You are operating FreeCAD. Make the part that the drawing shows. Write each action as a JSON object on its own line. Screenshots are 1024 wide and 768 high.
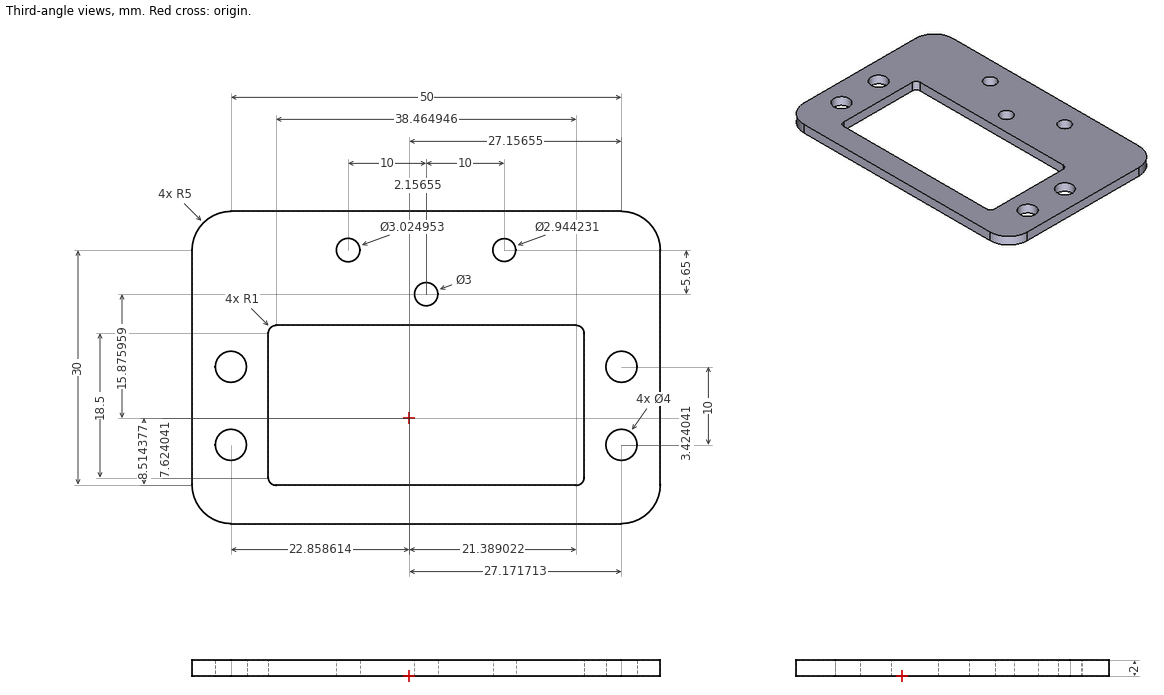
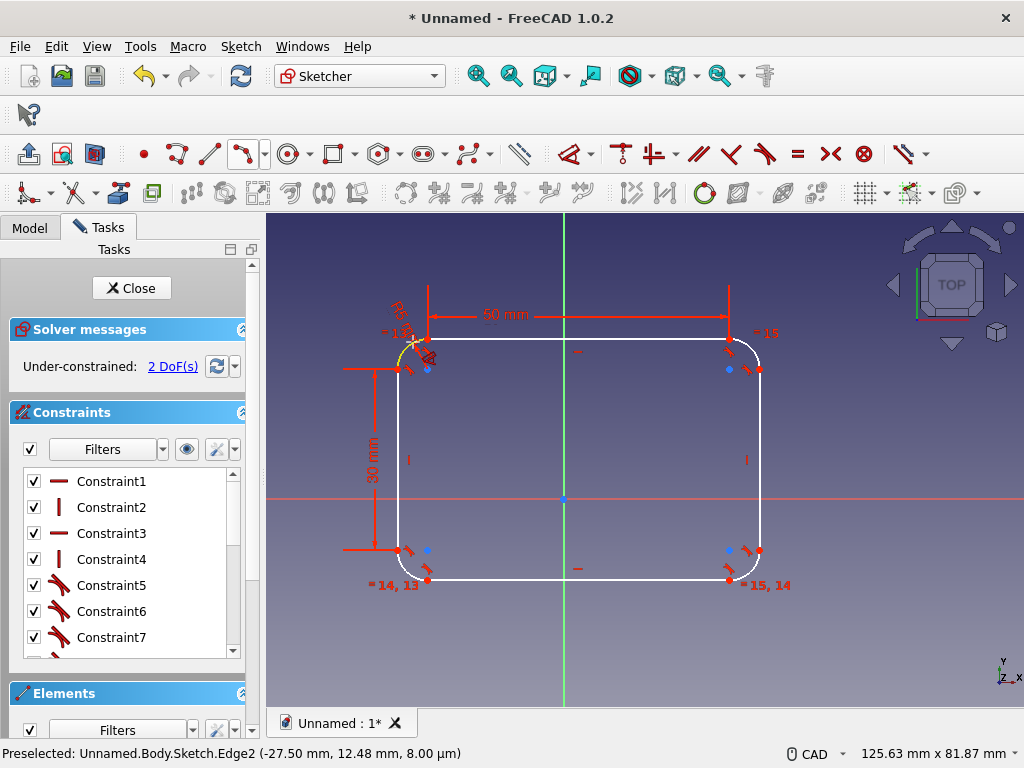
{"action": "left_click", "coordinate": [729, 339]}
{"action": "left_click", "coordinate": [647, 305]}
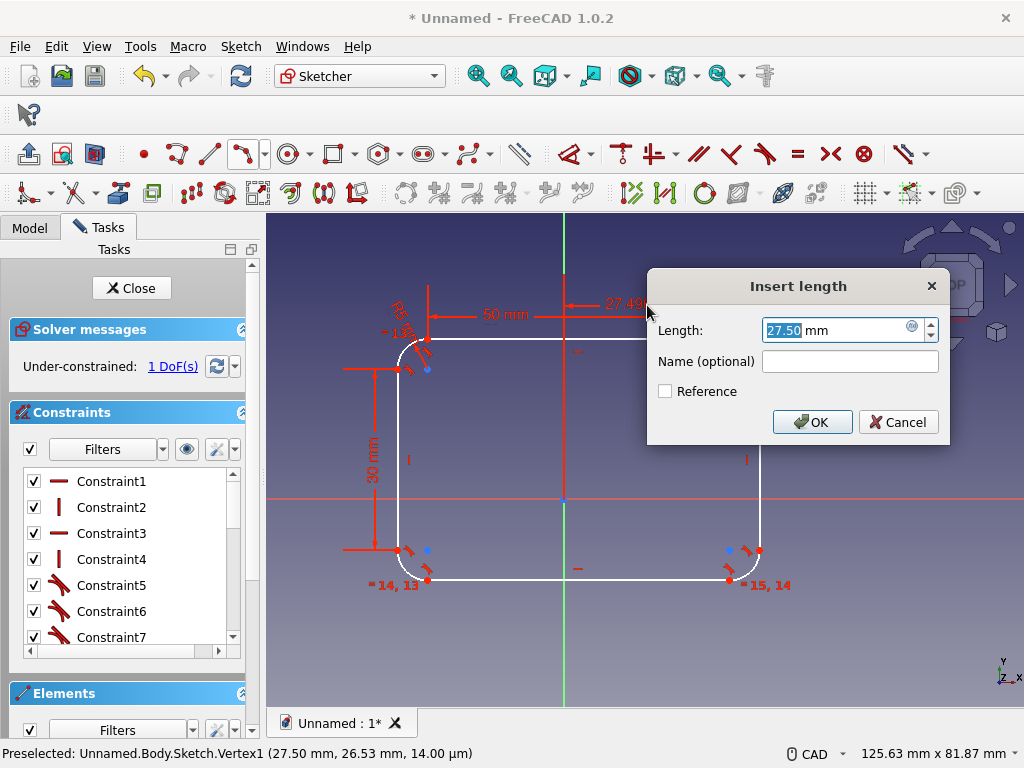
{"action": "type", "text": "27.15655"}
{"action": "key", "text": "Return"}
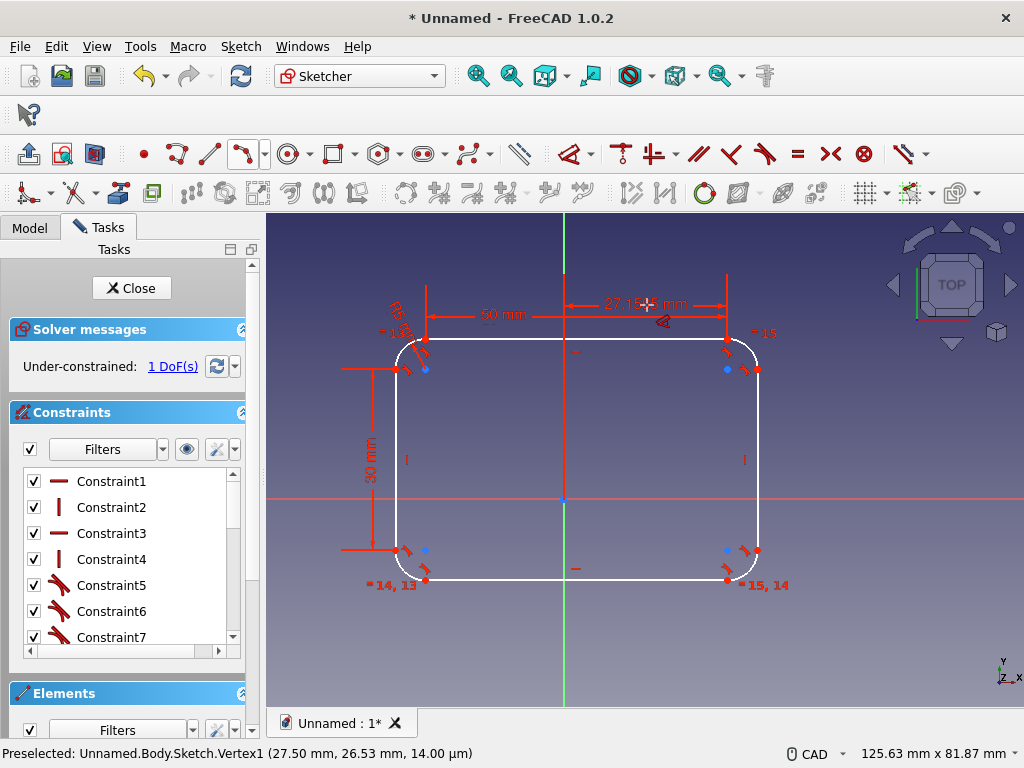
{"action": "left_click", "coordinate": [396, 550]}
{"action": "left_click", "coordinate": [362, 525]}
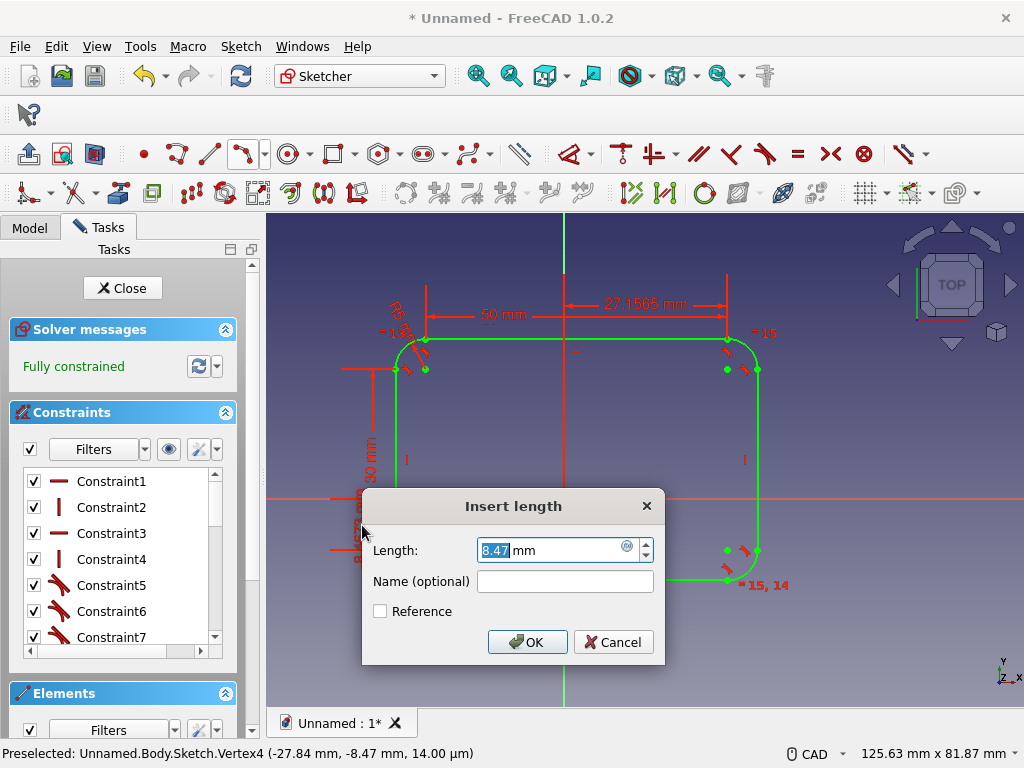
{"action": "type", "text": "8.514377"}
{"action": "key", "text": "Return"}
{"action": "key", "text": "Escape"}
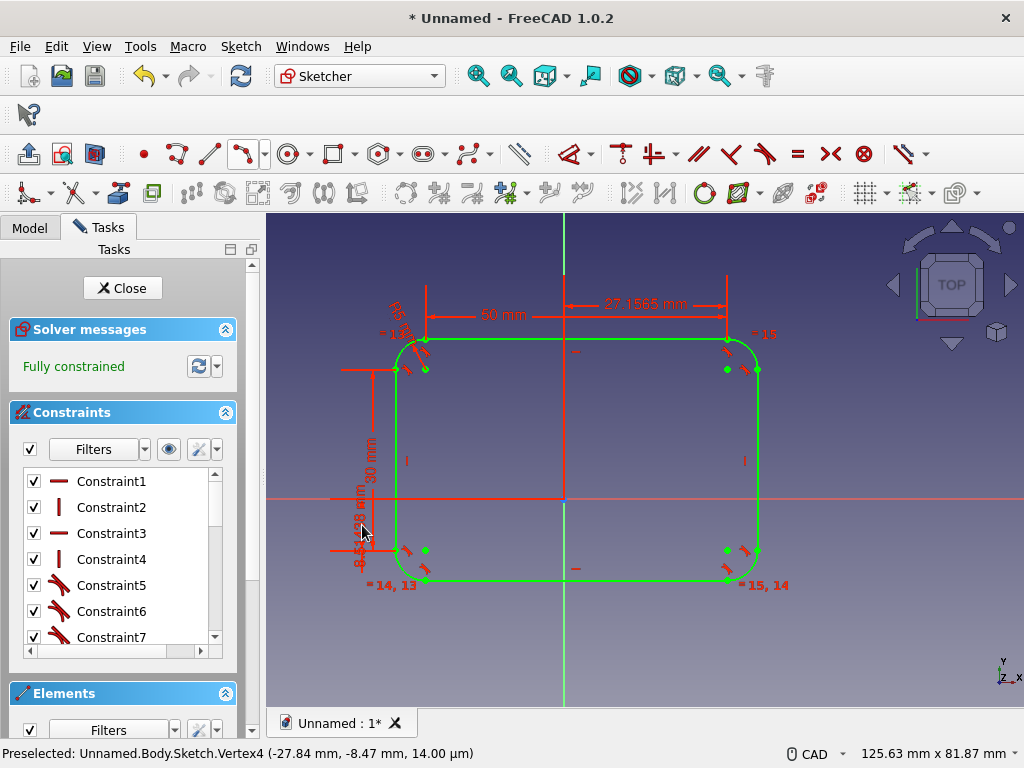
{"action": "left_click", "coordinate": [123, 288]}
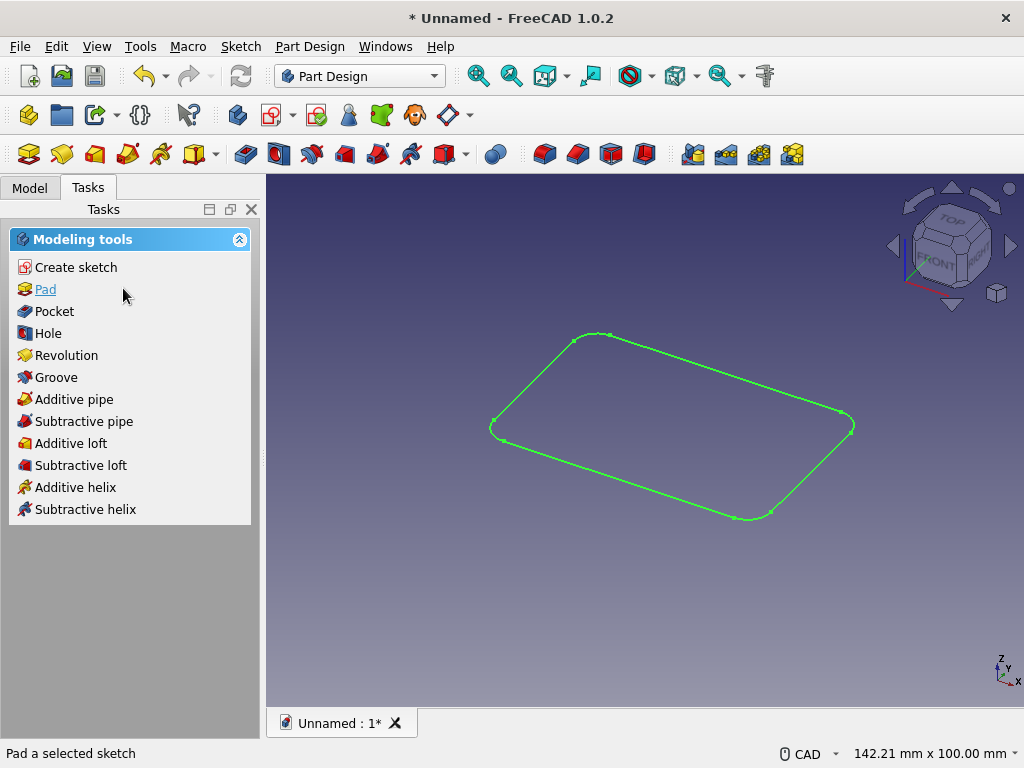
{"action": "left_click", "coordinate": [29, 154]}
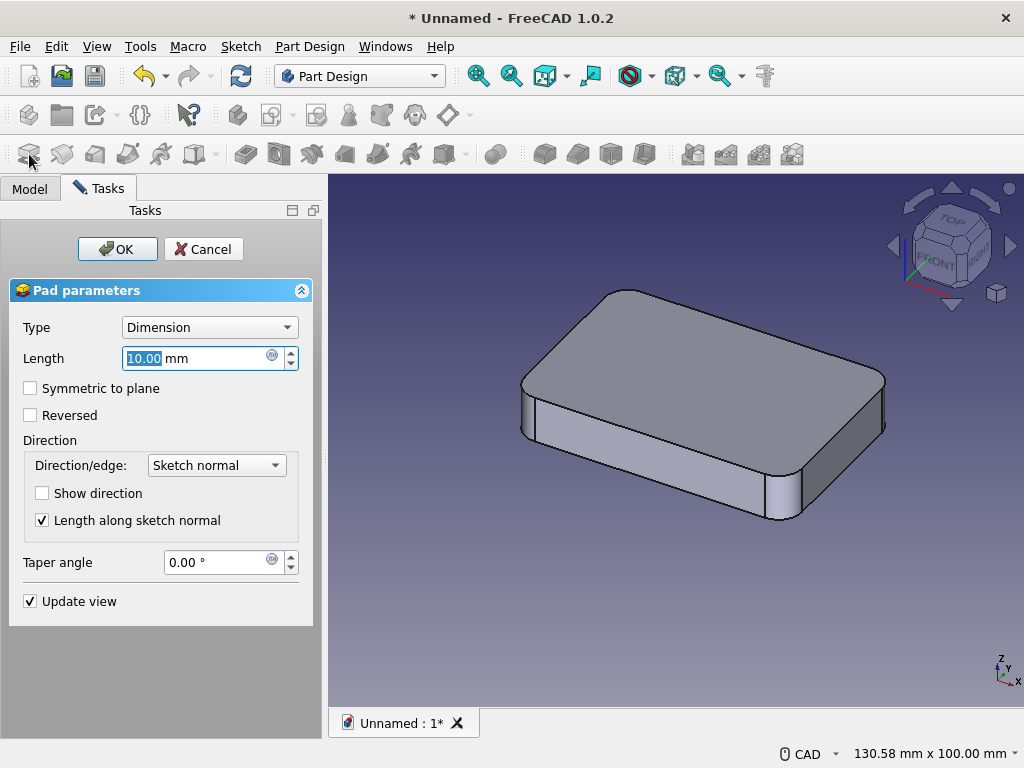
{"action": "type", "text": "2"}
{"action": "key", "text": "Tab"}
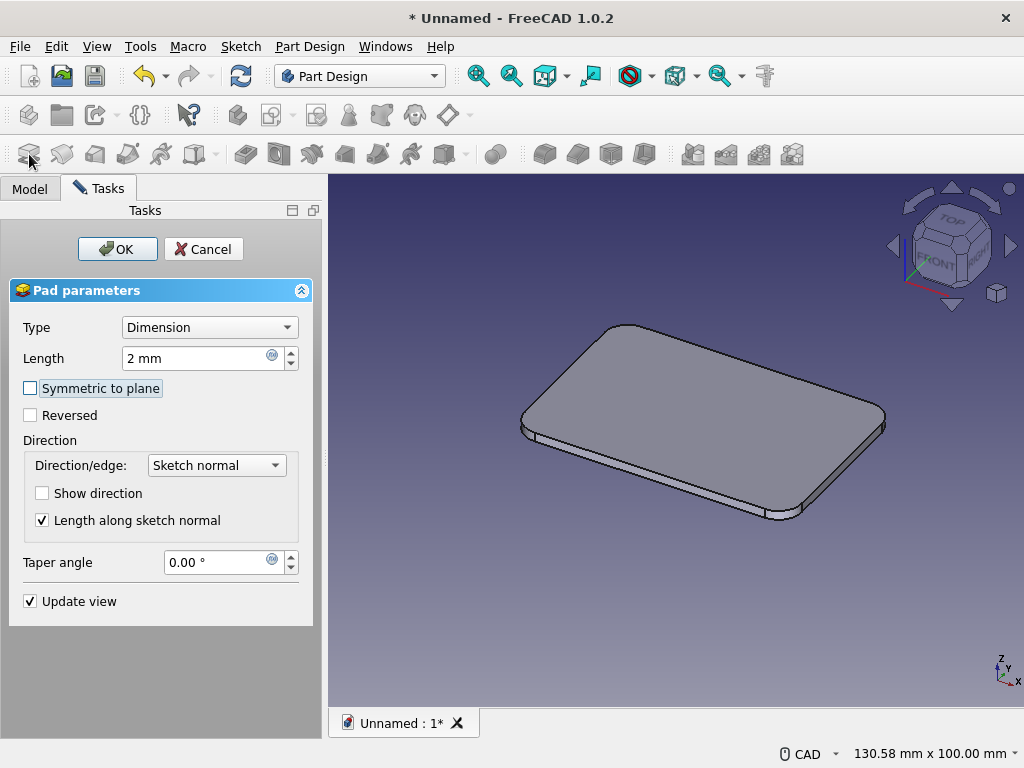
{"action": "left_click", "coordinate": [118, 249]}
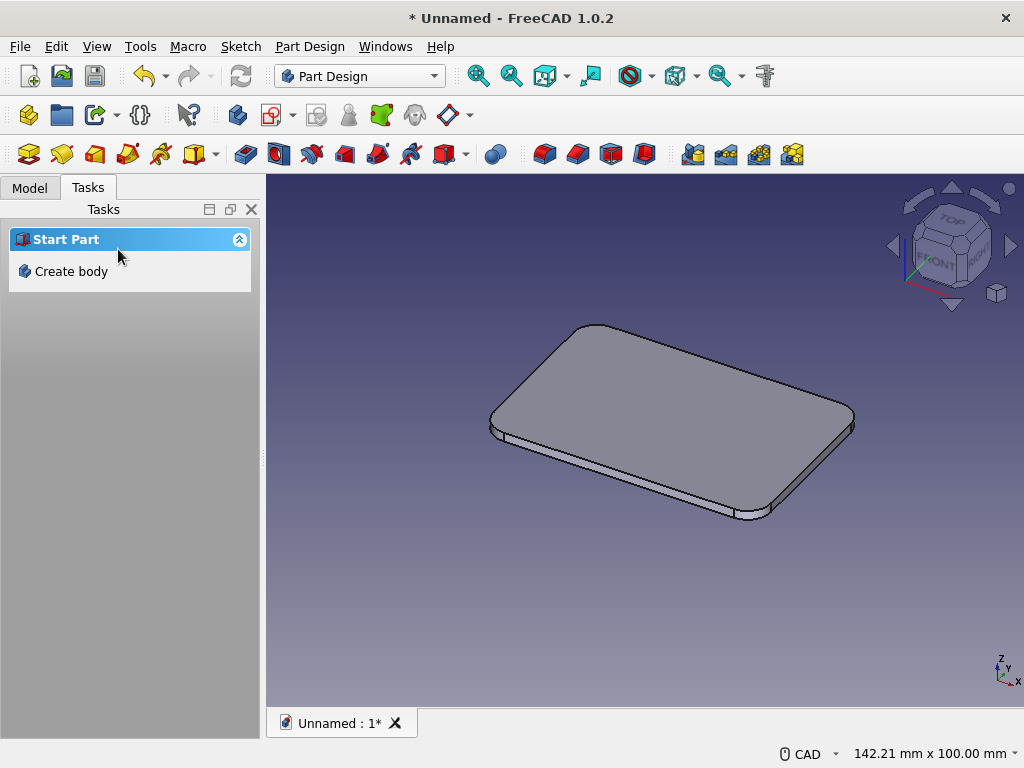
{"action": "left_click", "coordinate": [712, 430]}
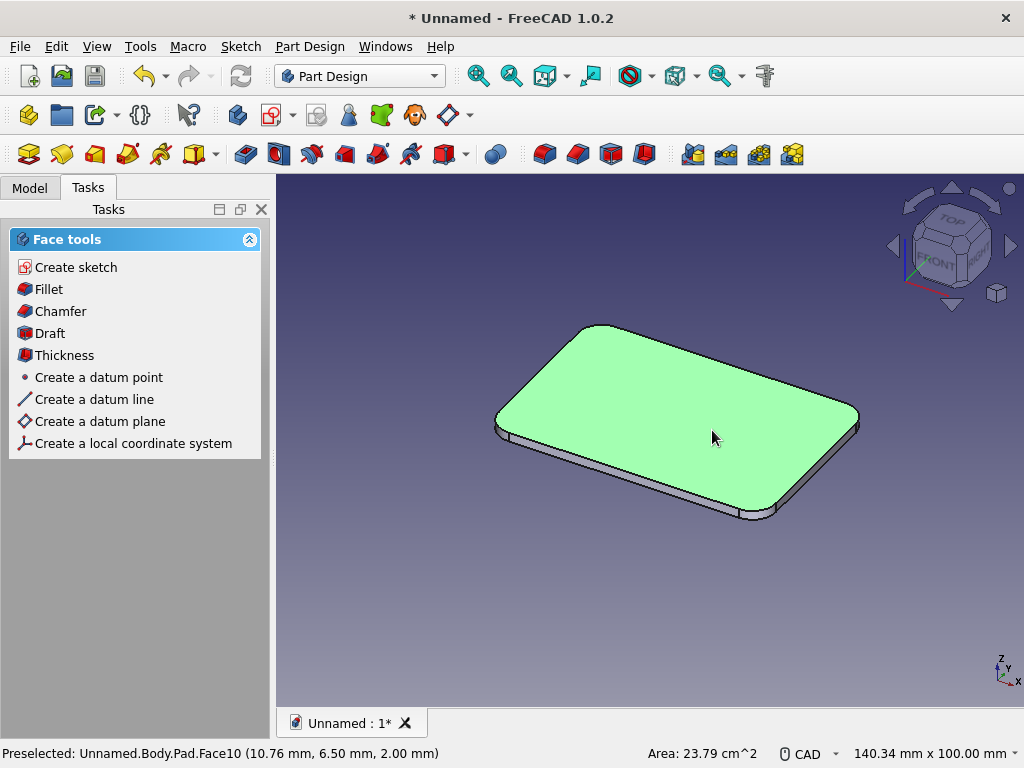
{"action": "left_click", "coordinate": [270, 116]}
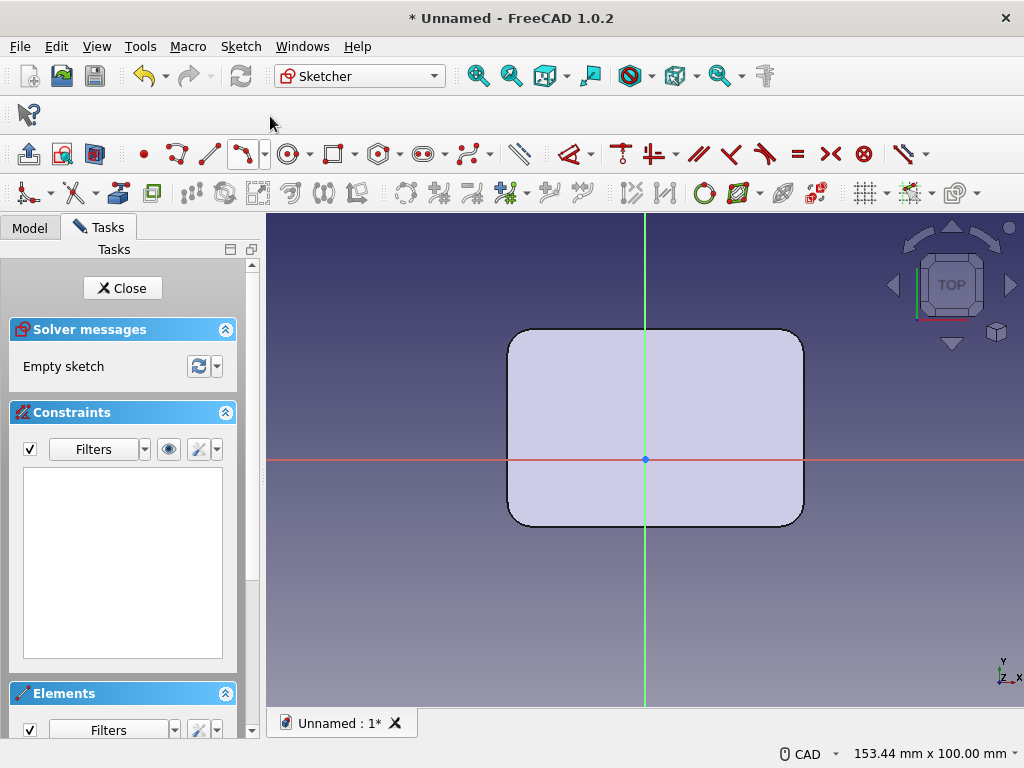
{"action": "scroll", "coordinate": [752, 442], "scroll_direction": "up", "scroll_amount": 3}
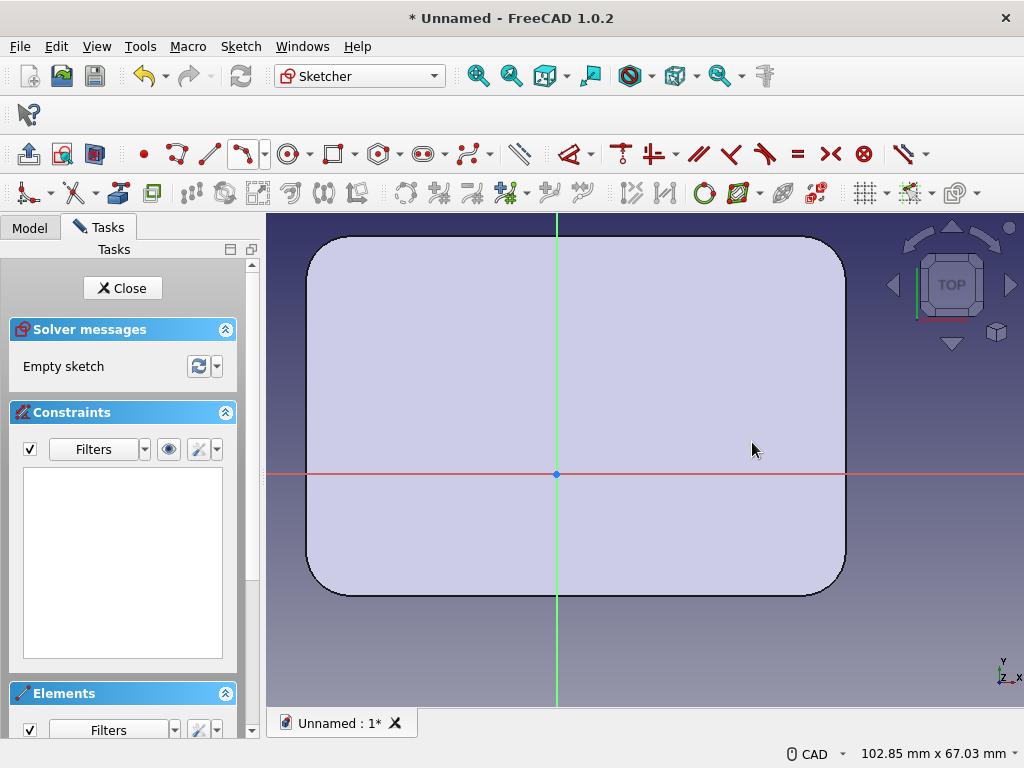
{"action": "left_click", "coordinate": [210, 154]}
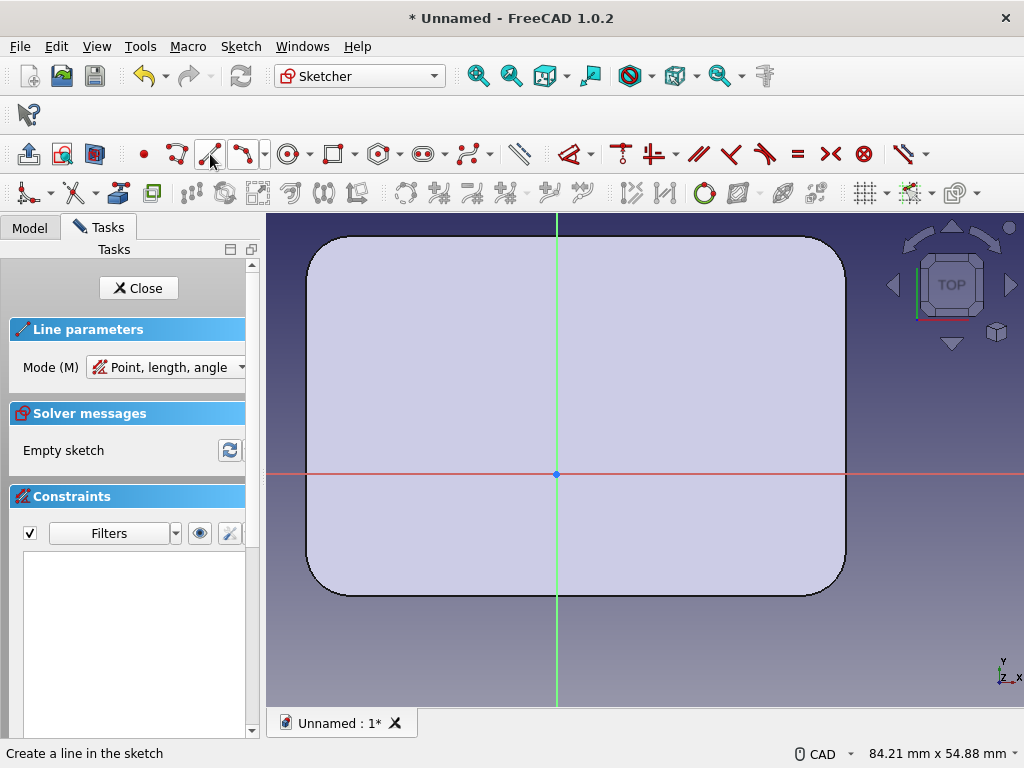
{"action": "left_click", "coordinate": [749, 368]}
{"action": "left_click", "coordinate": [403, 368]}